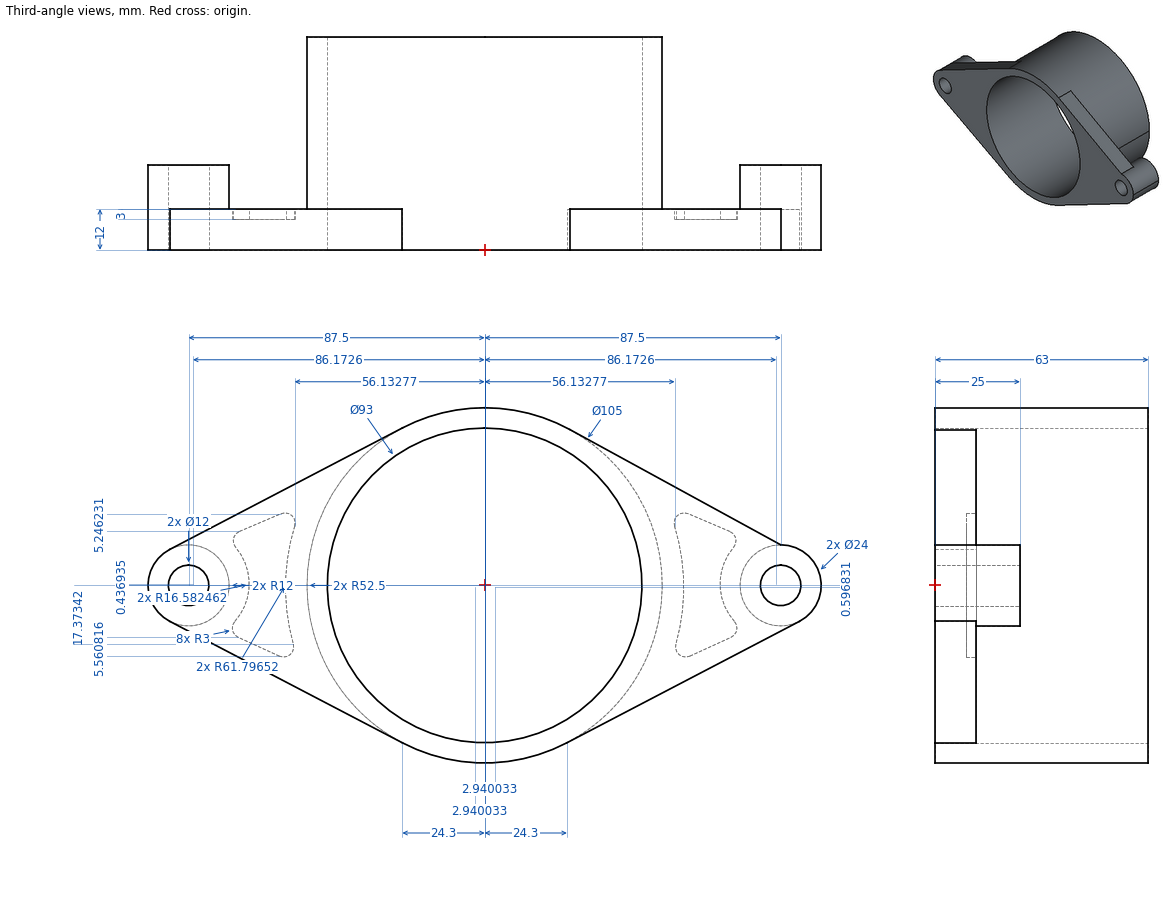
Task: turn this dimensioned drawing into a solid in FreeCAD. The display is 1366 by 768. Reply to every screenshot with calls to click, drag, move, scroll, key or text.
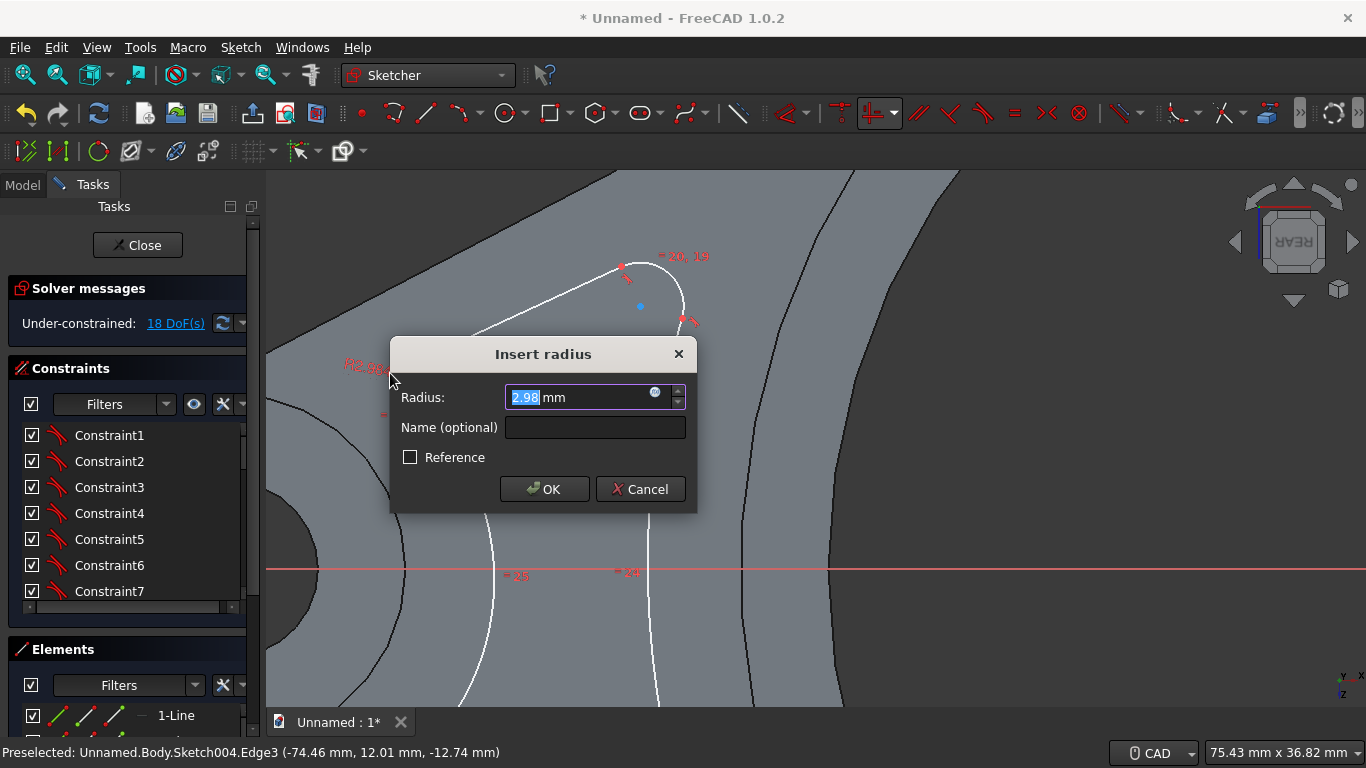
text(3)
key(Return)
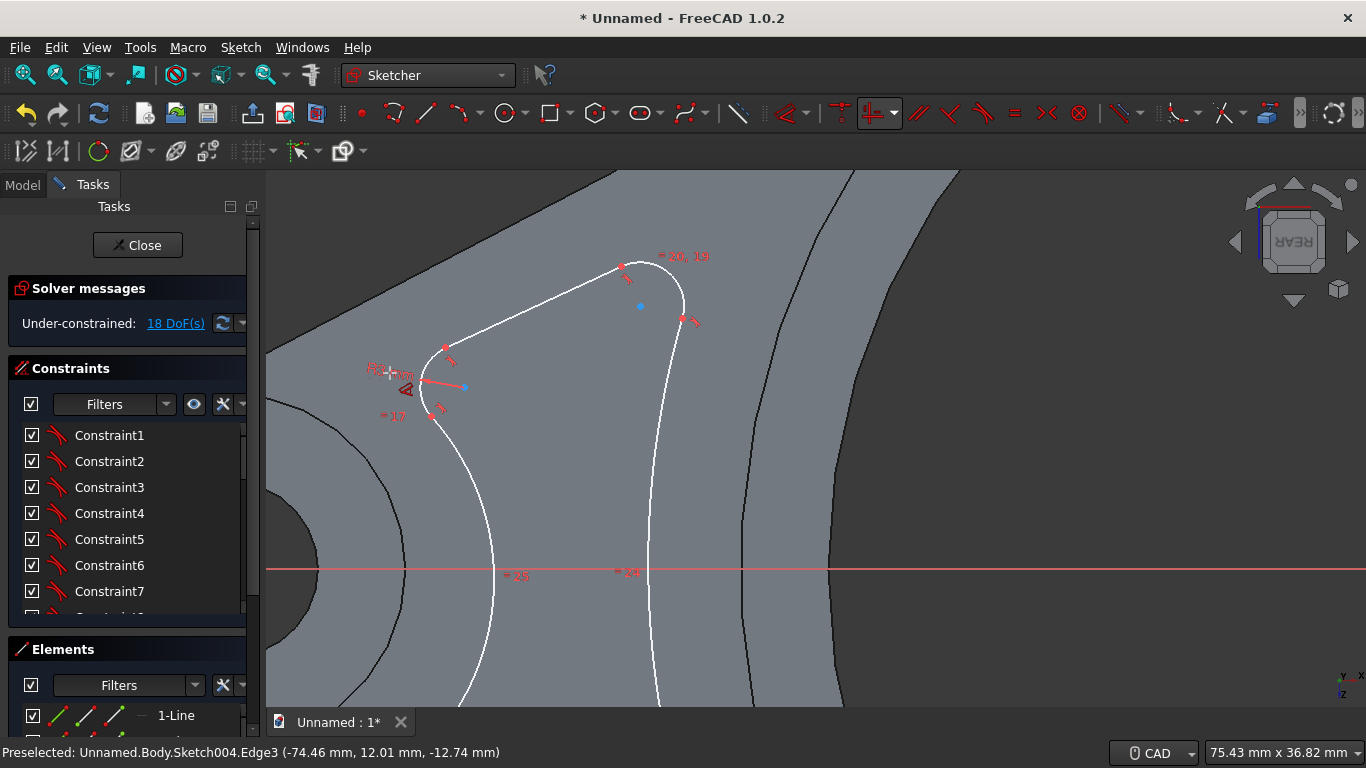
click(485, 646)
click(516, 655)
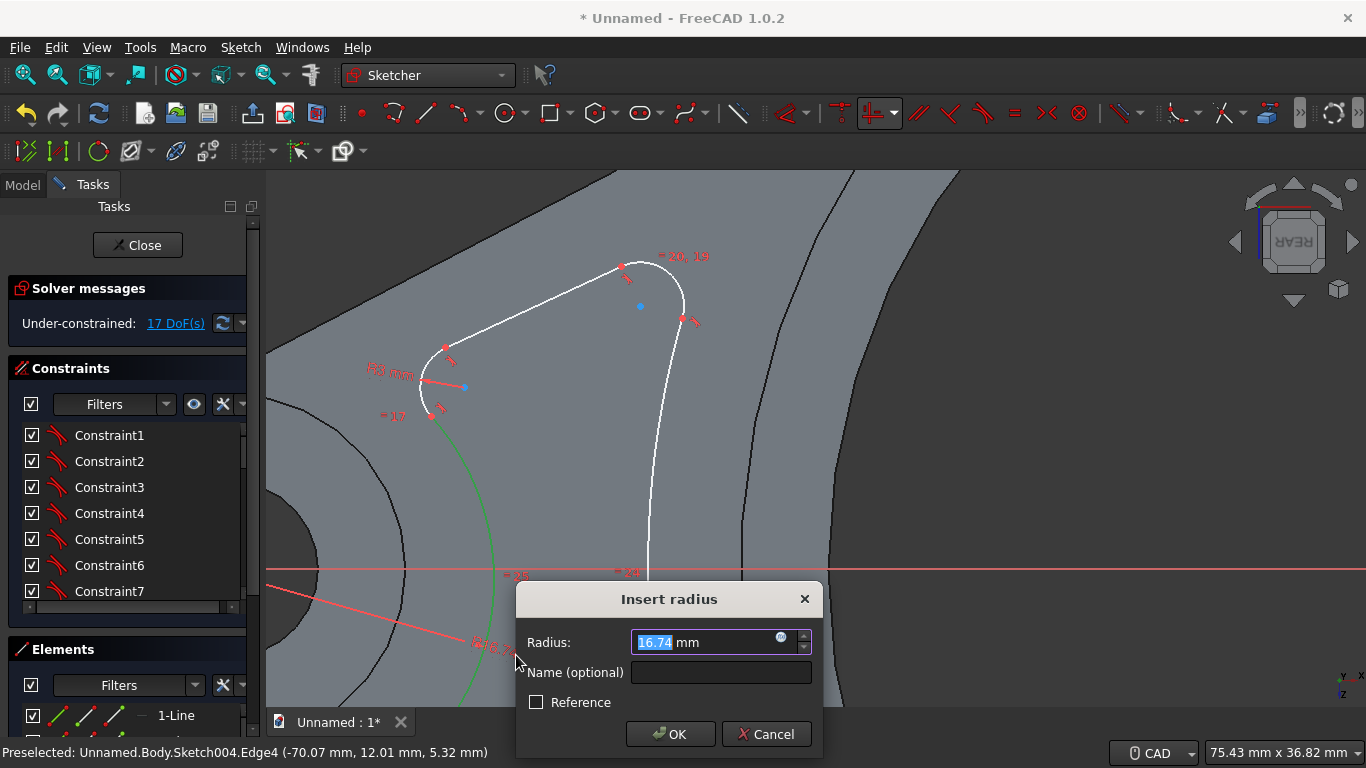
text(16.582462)
key(Return)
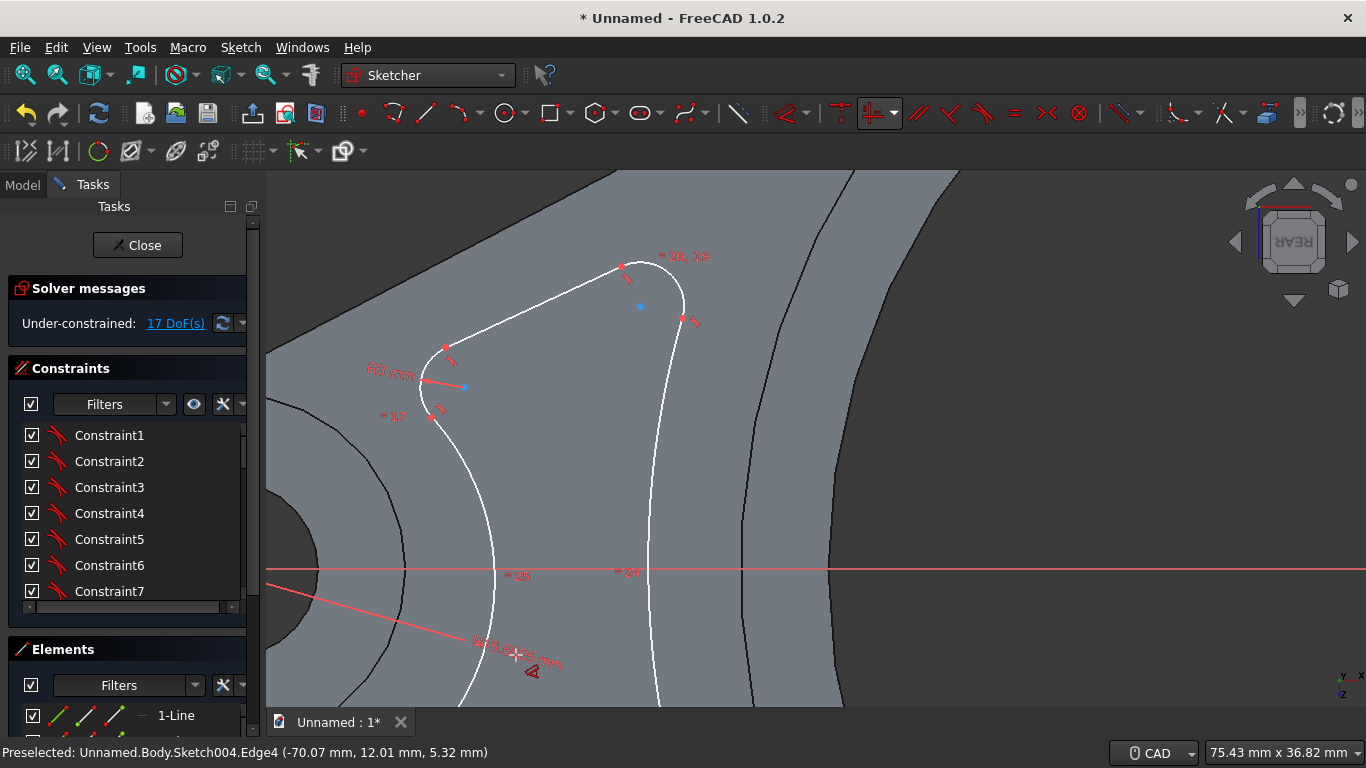
click(653, 470)
click(621, 467)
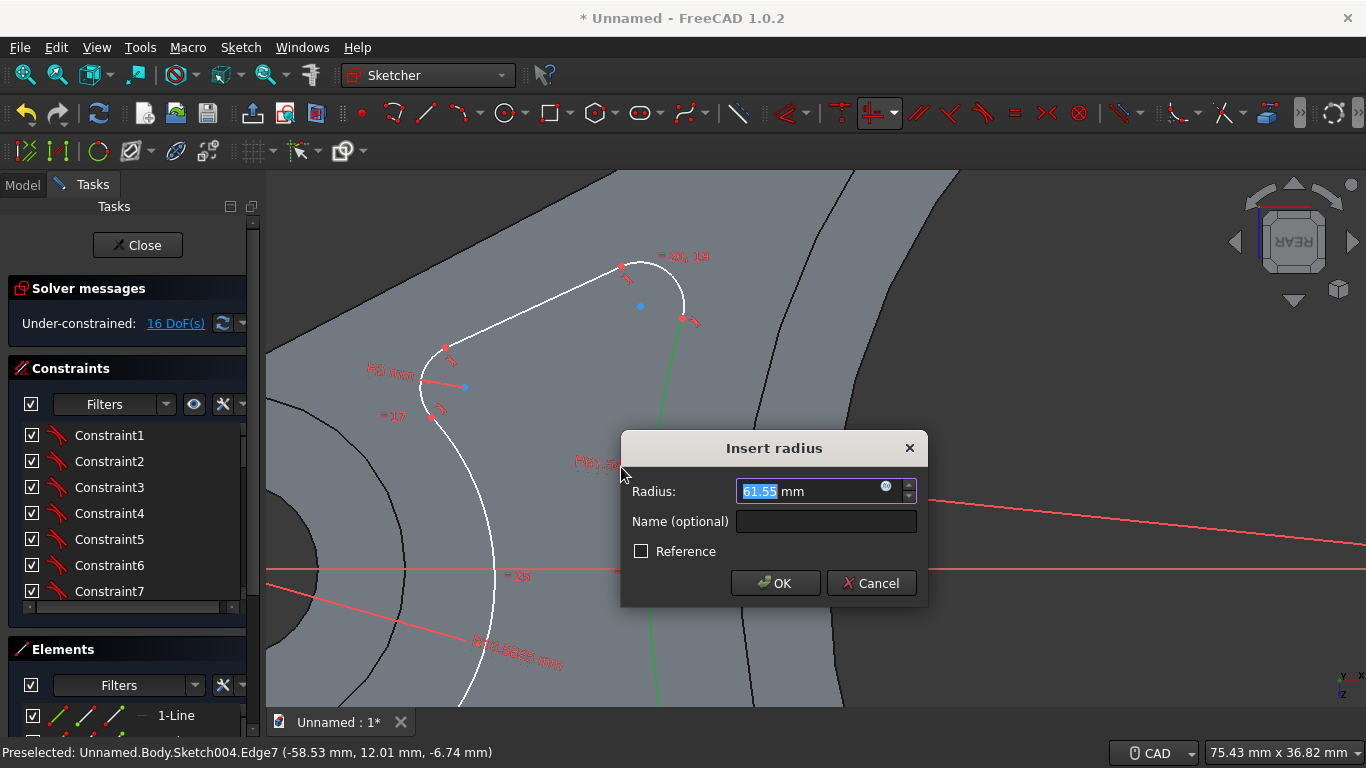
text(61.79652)
key(Return)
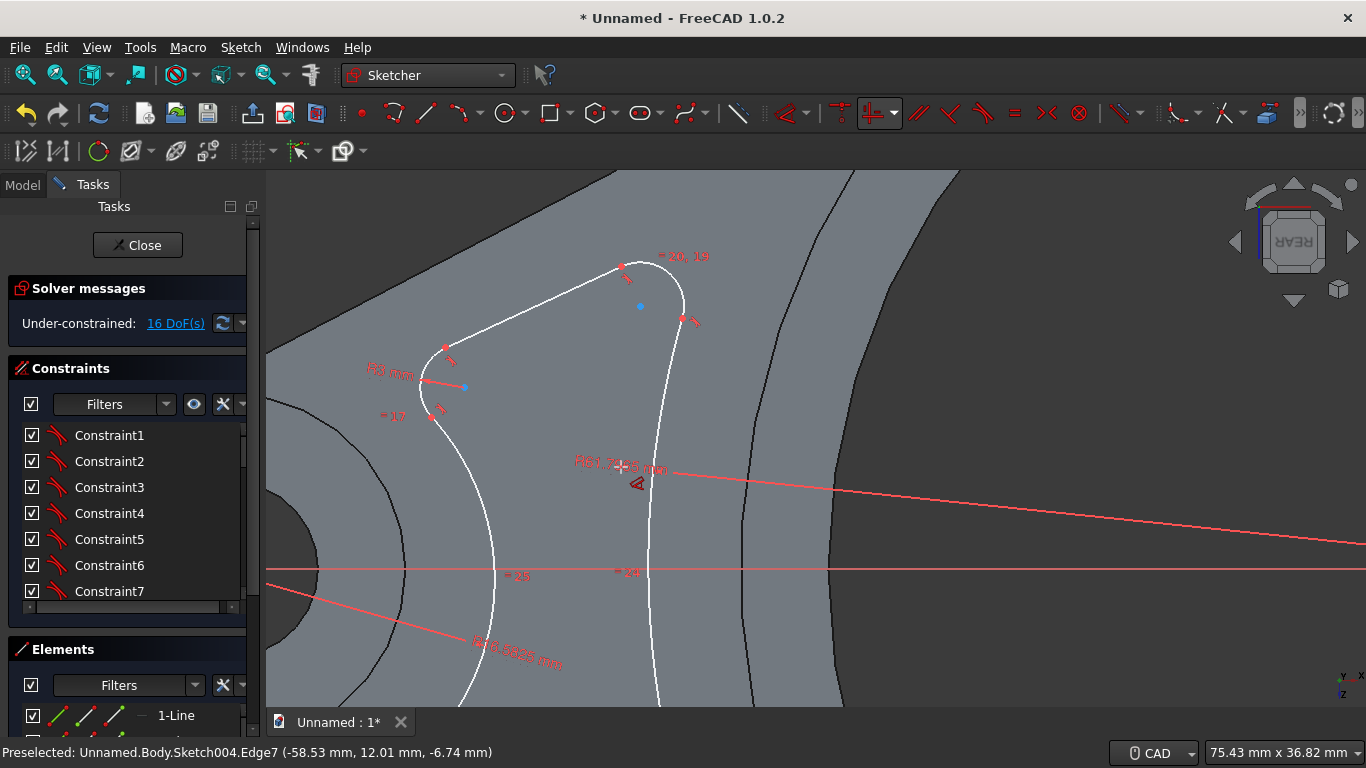
scroll(420, 381, down, 6)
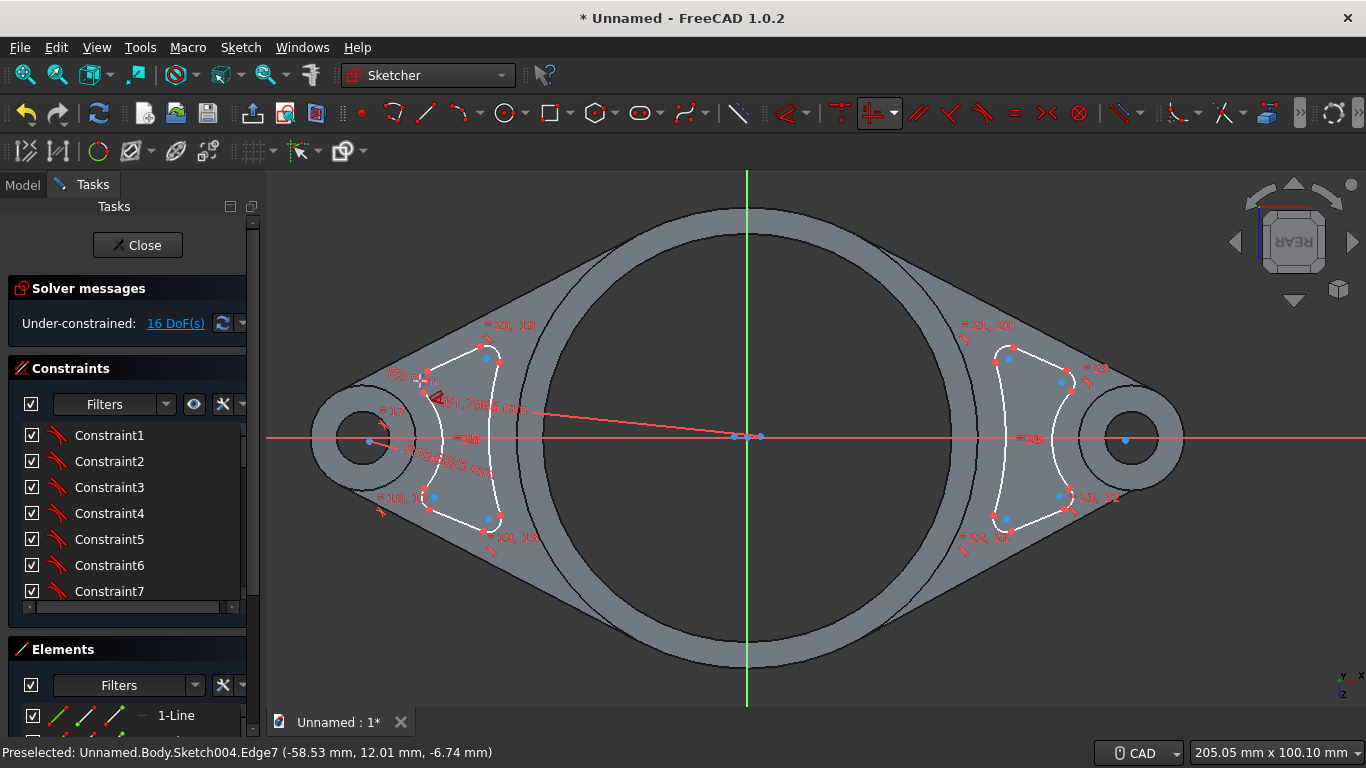
click(370, 441)
click(559, 475)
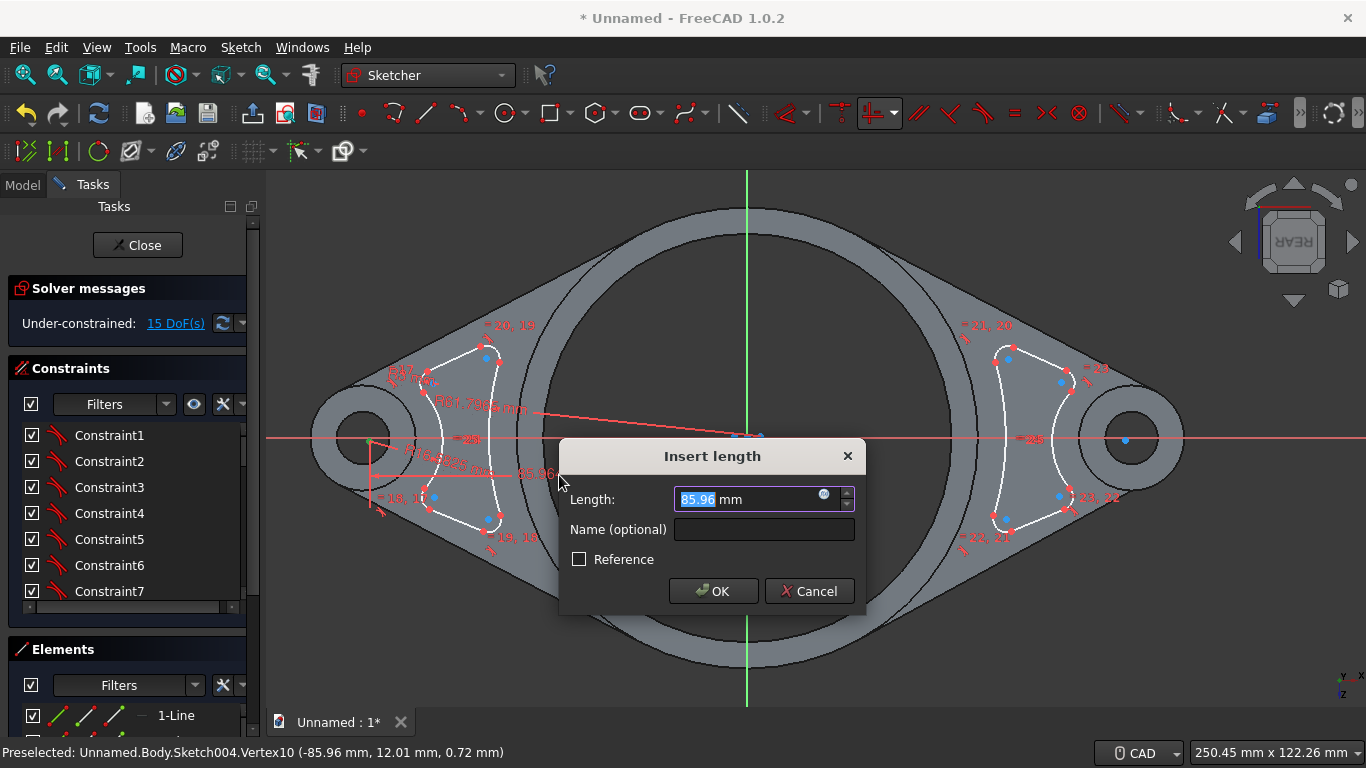
text(86.1726)
key(Return)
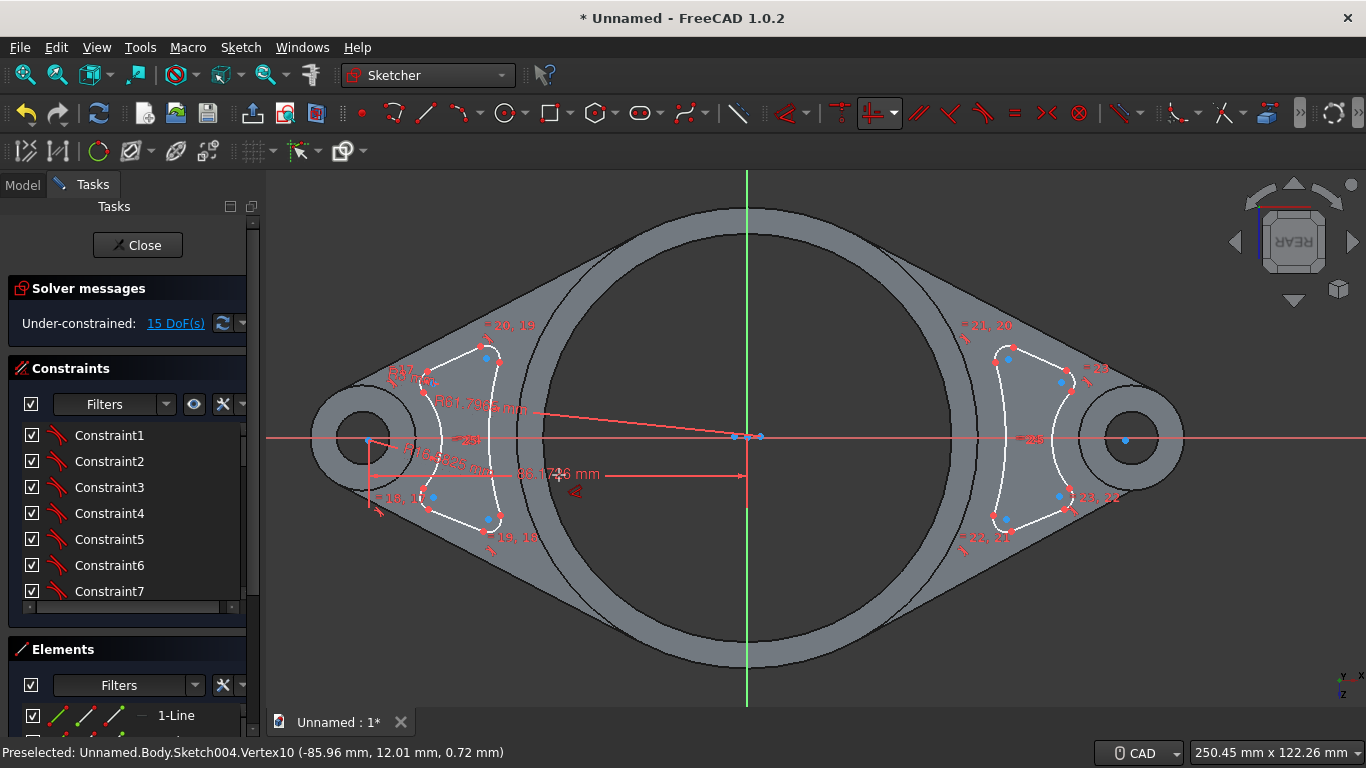
click(1125, 441)
click(936, 475)